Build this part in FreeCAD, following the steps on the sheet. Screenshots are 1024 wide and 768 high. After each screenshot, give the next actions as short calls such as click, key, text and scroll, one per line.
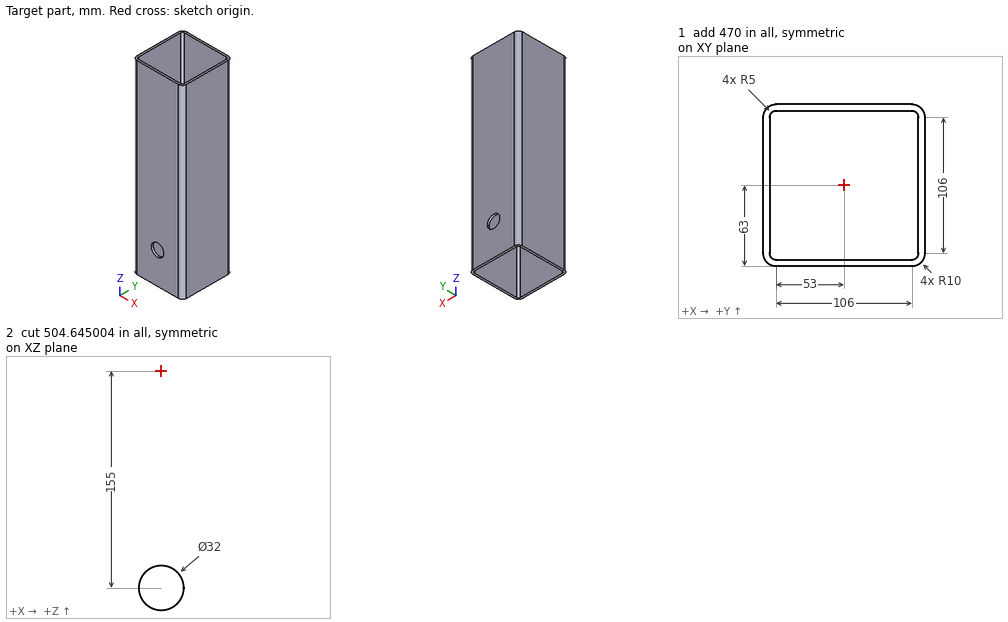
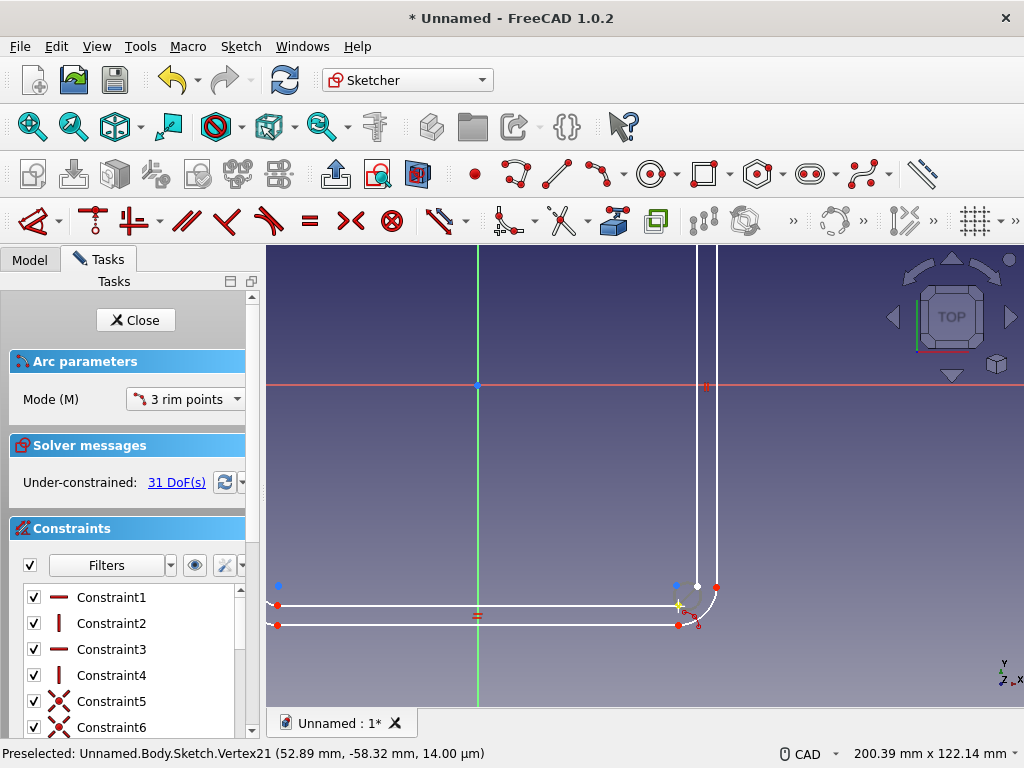
scroll(692, 599, up, 6)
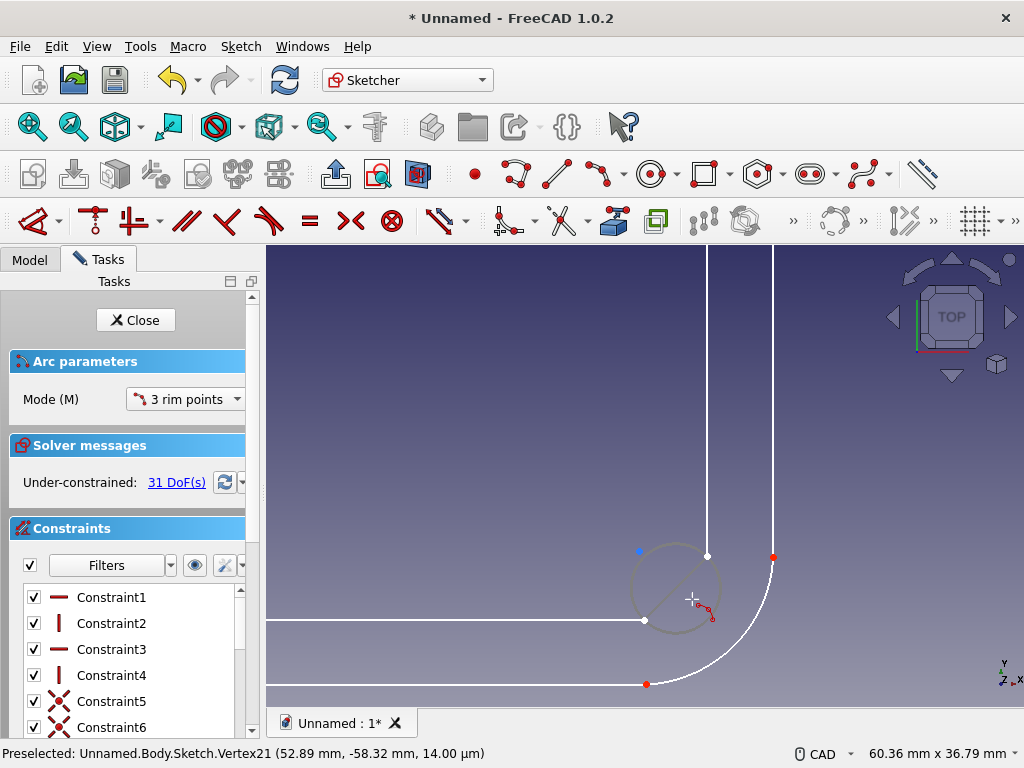
click(690, 598)
key(Escape)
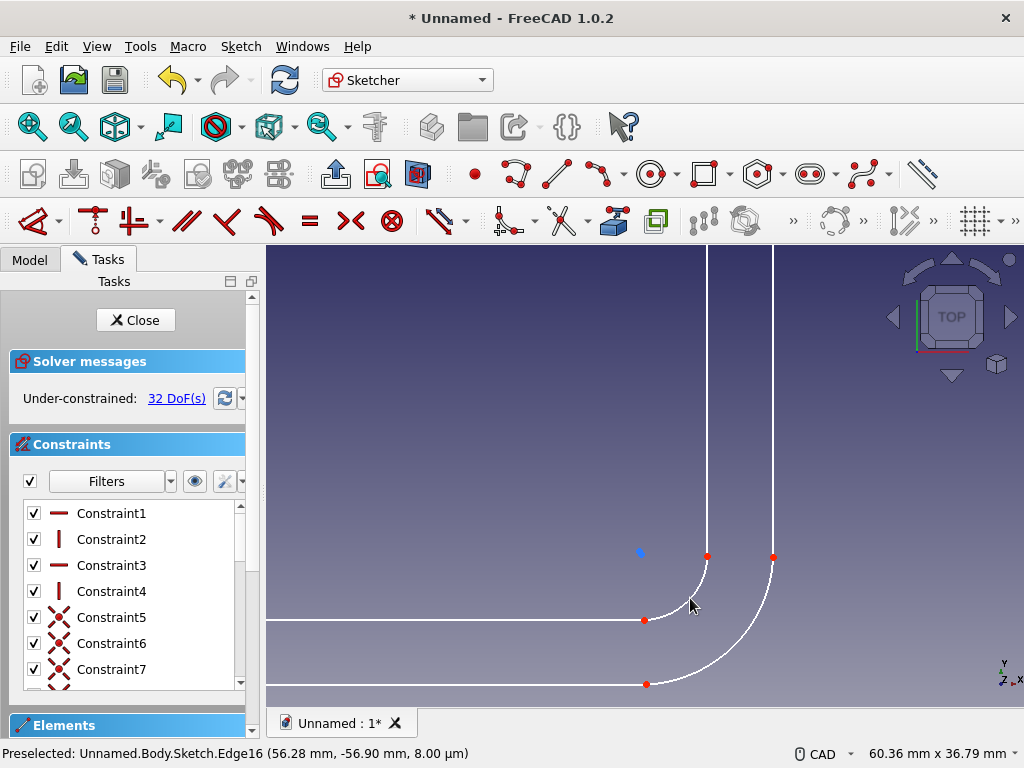
scroll(695, 593, down, 9)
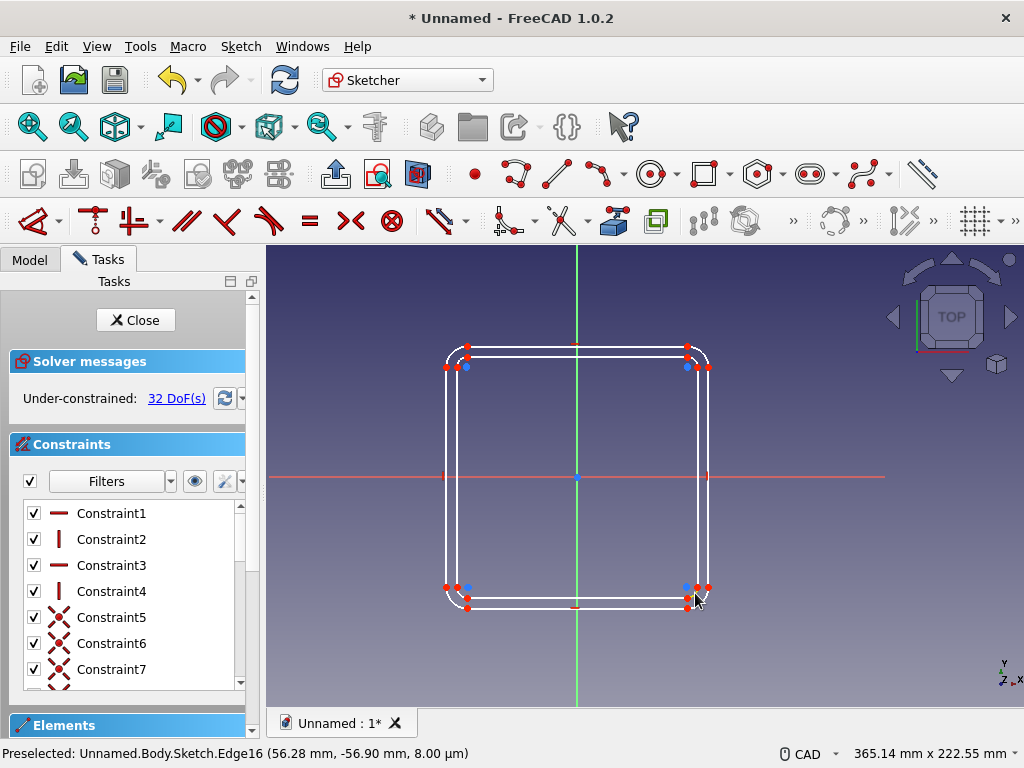
scroll(533, 609, up, 2)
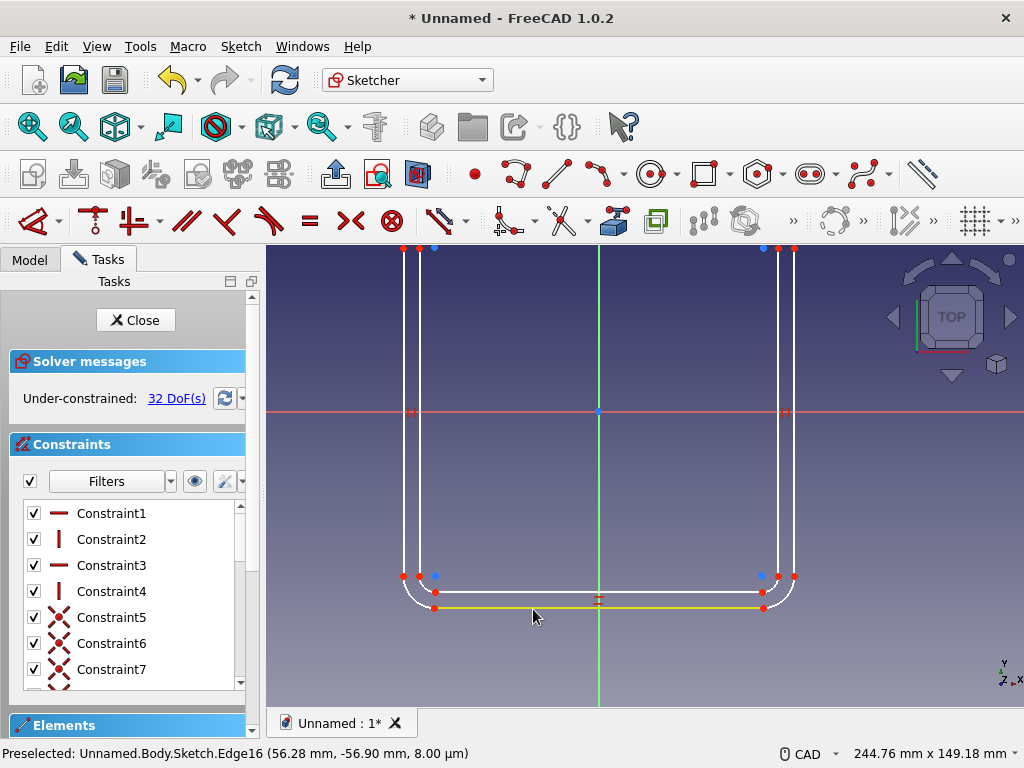
click(533, 608)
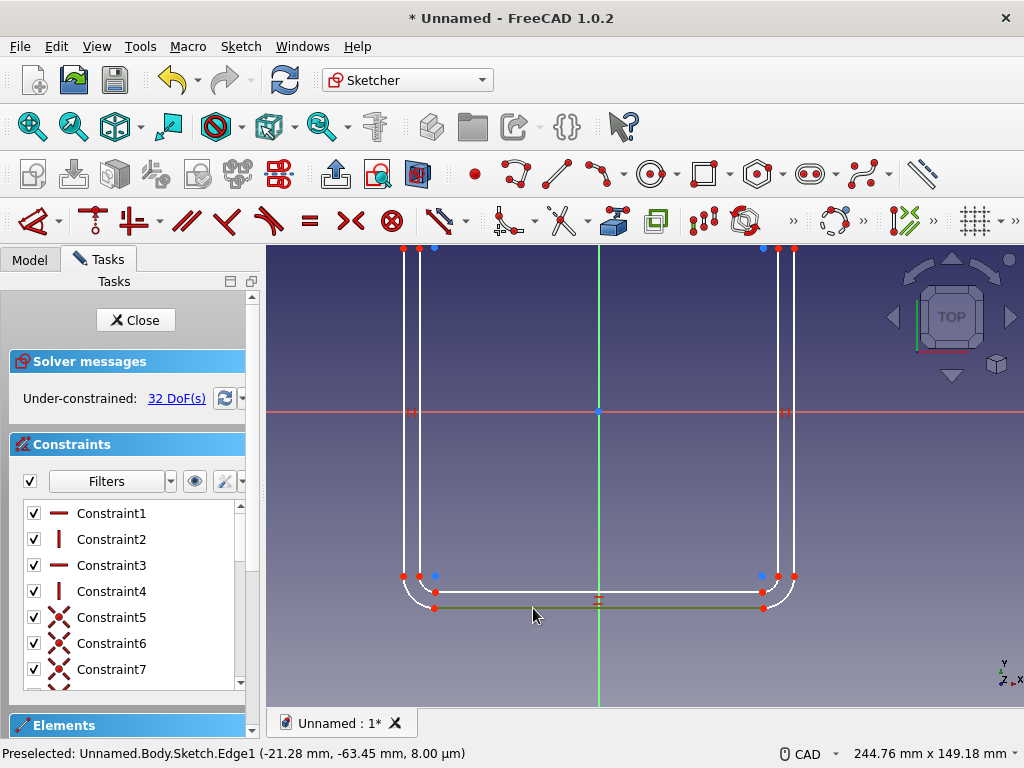
click(777, 604)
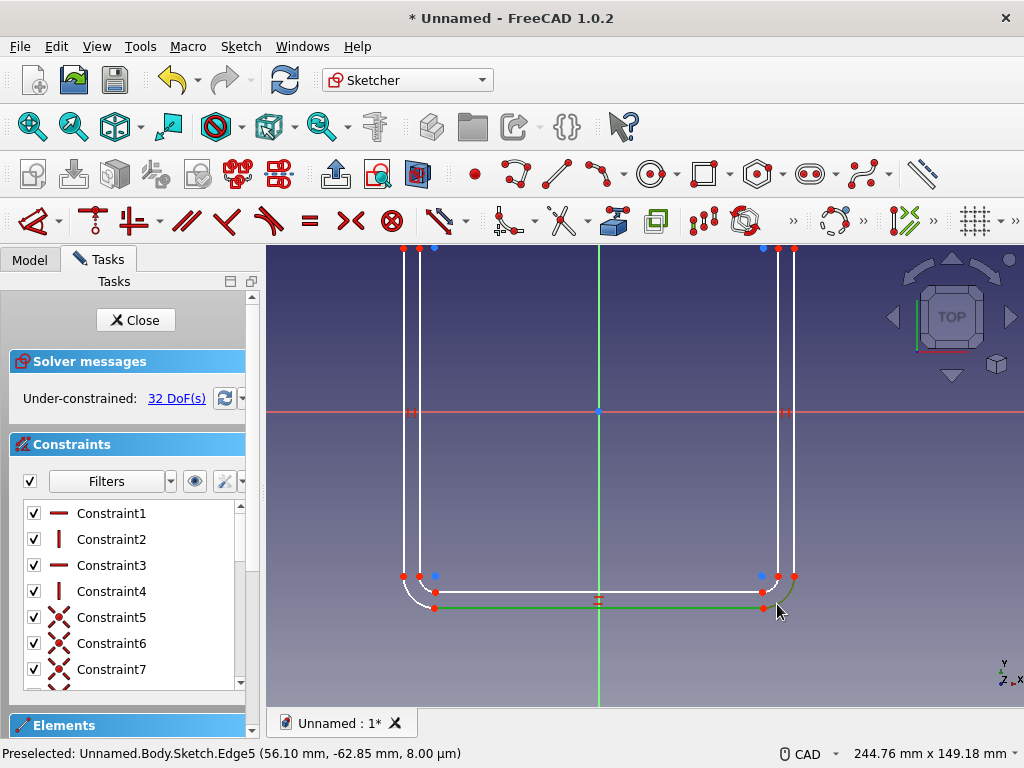
click(269, 222)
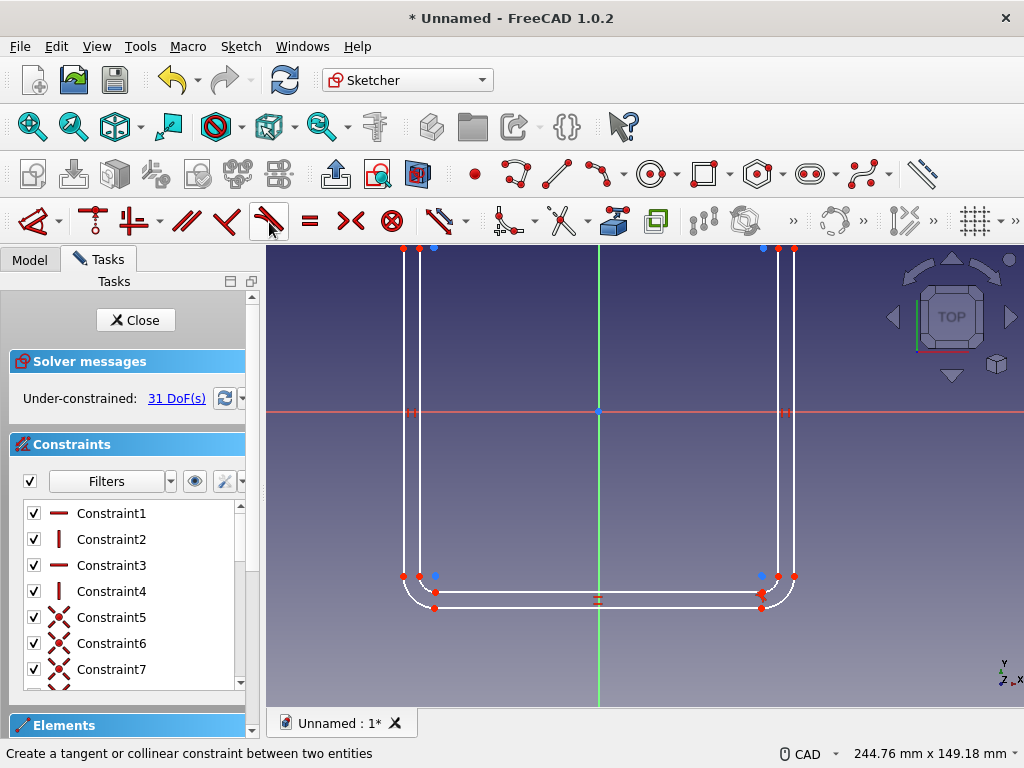
click(533, 608)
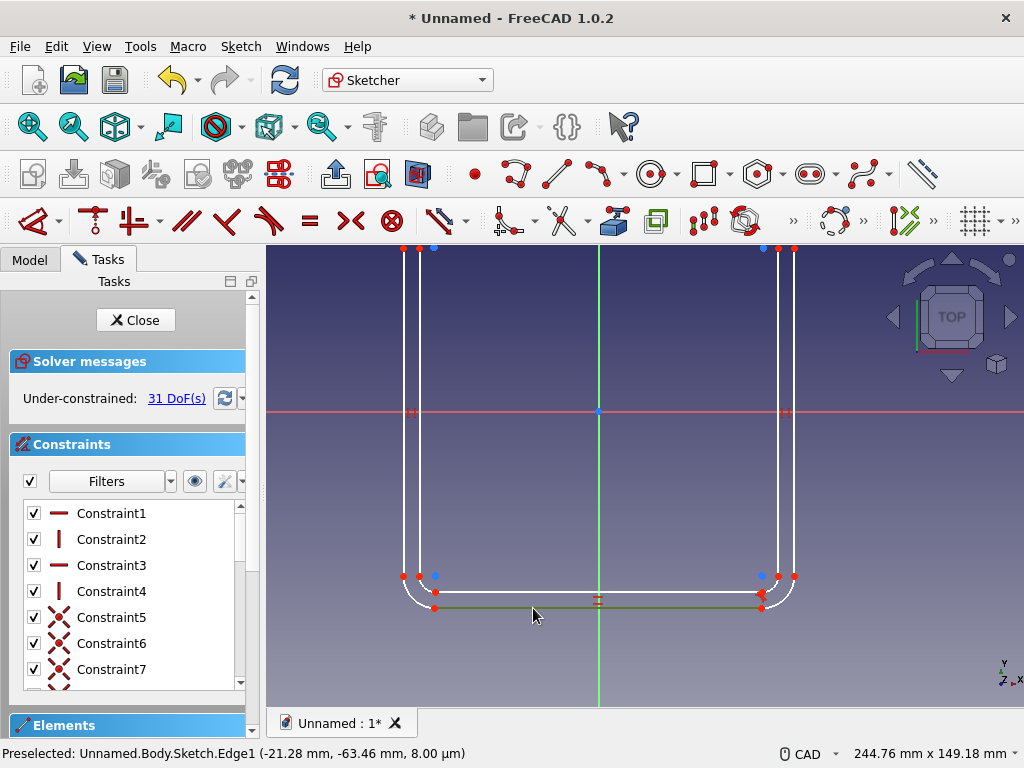
click(407, 591)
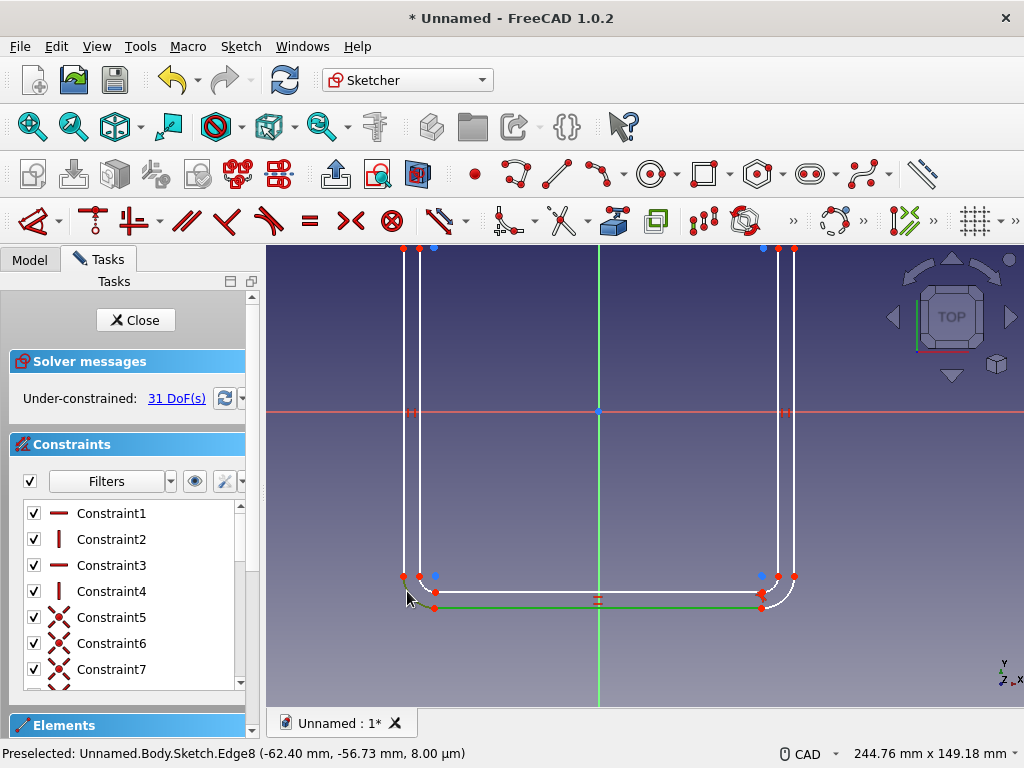
click(269, 222)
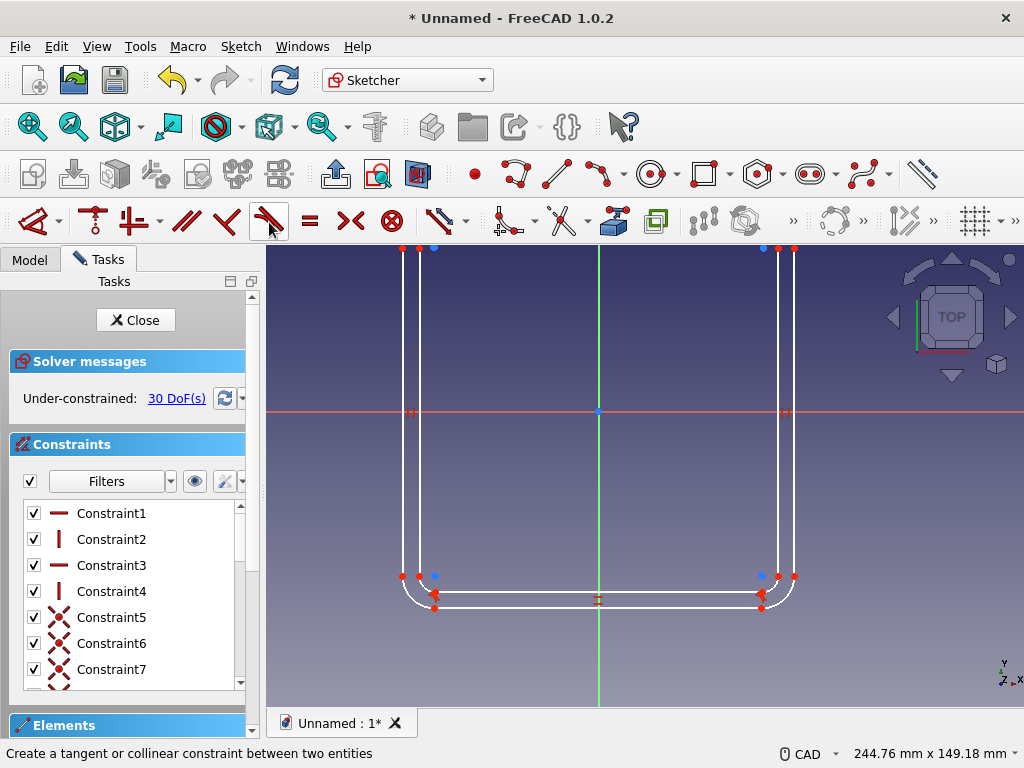
click(794, 478)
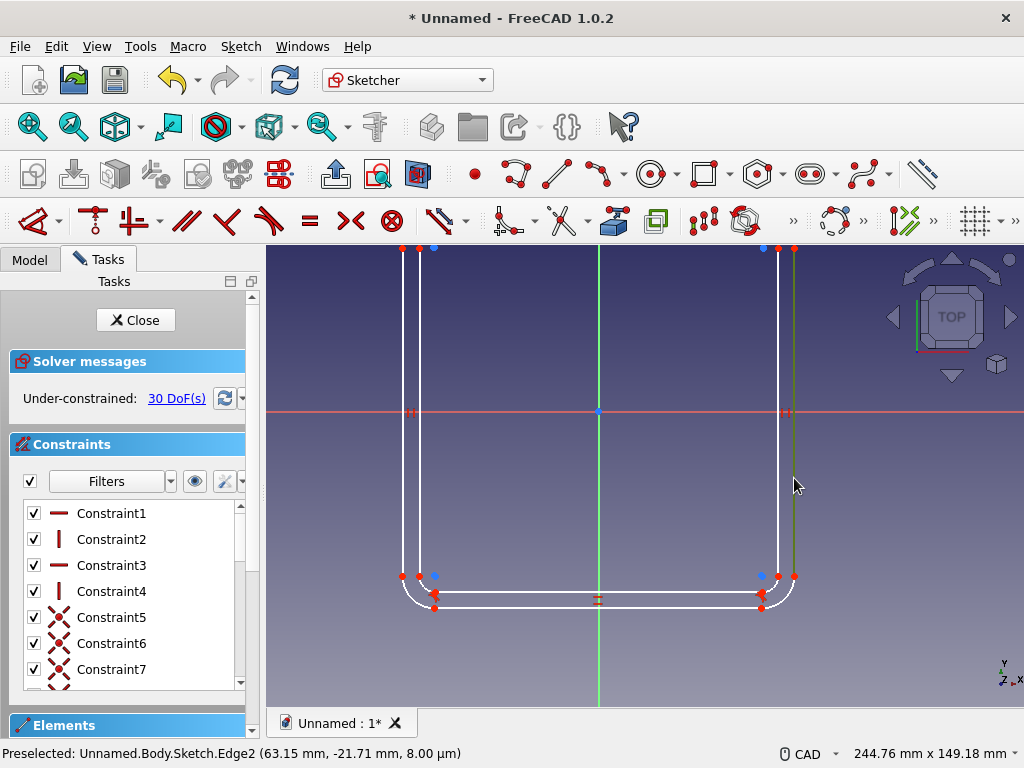
click(776, 605)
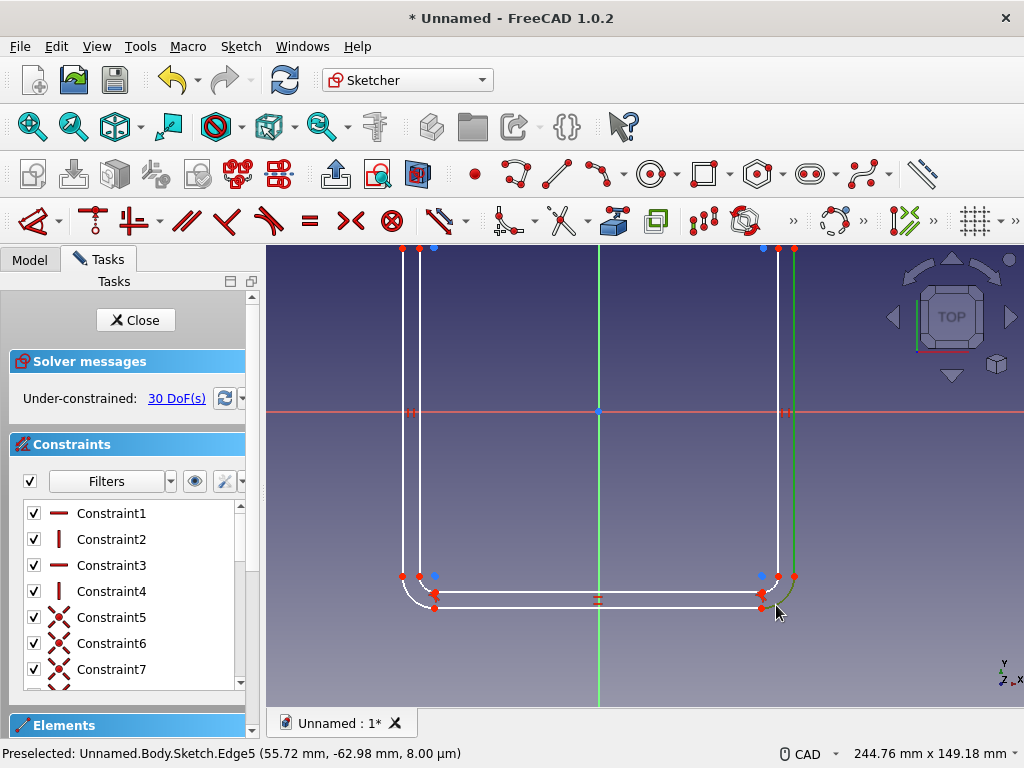
key(t)